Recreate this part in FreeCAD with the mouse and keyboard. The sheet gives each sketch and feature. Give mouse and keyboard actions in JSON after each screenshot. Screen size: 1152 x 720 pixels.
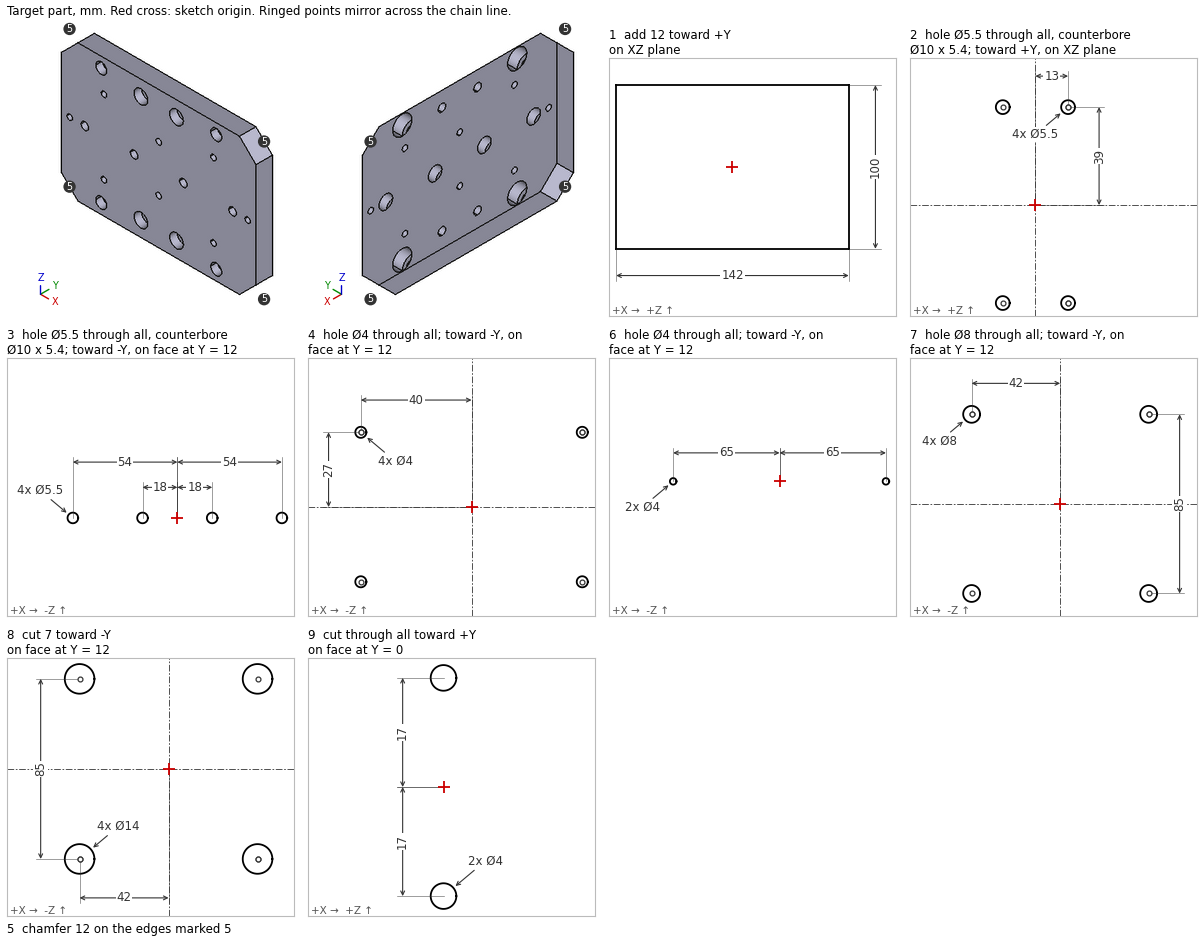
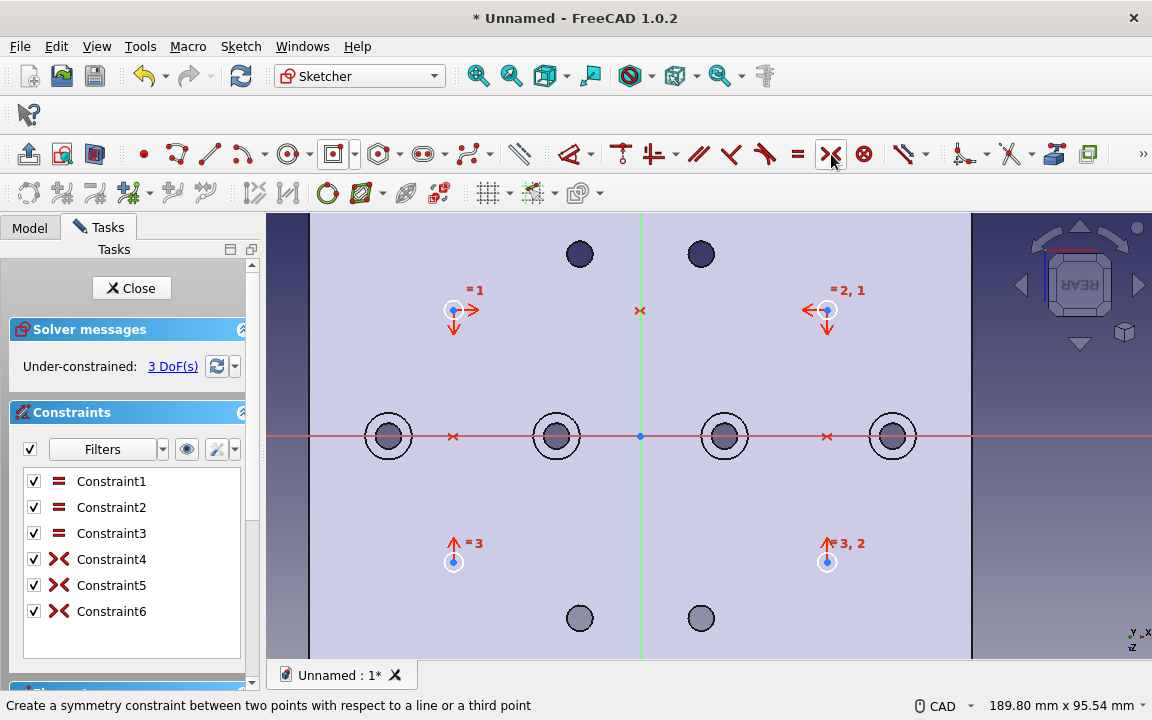
{"action": "left_click", "coordinate": [568, 154]}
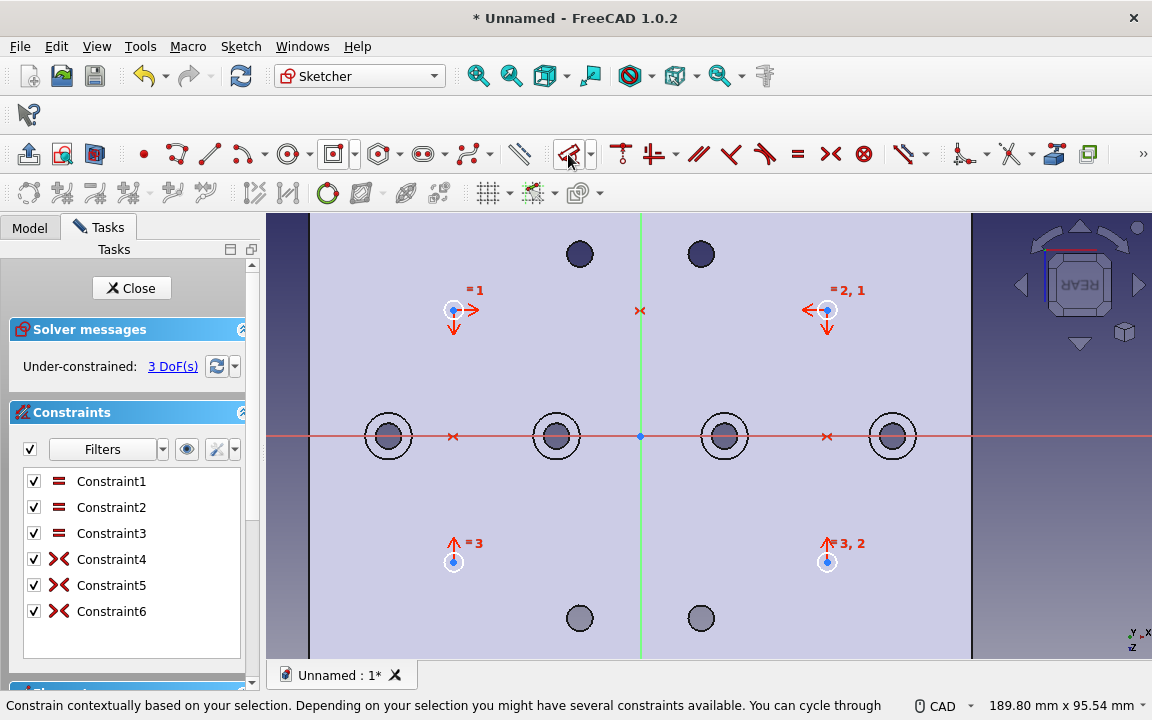
{"action": "scroll", "coordinate": [460, 303], "scroll_direction": "up", "scroll_amount": 4}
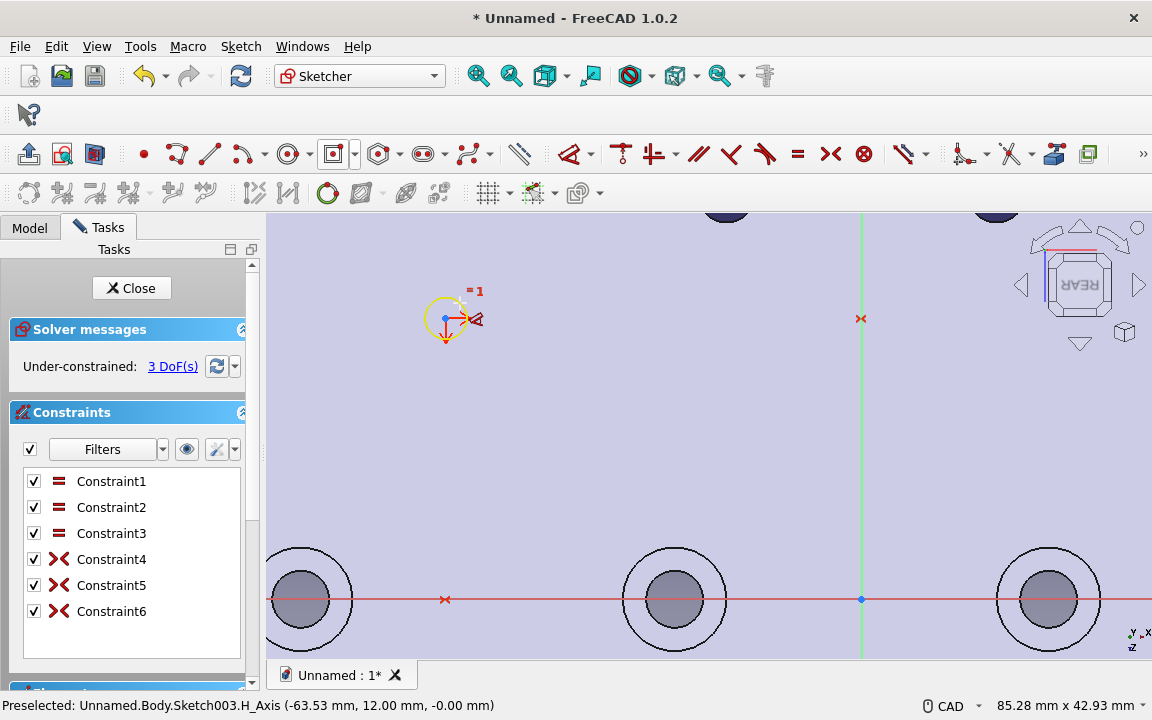
{"action": "left_click", "coordinate": [461, 304]}
{"action": "left_click", "coordinate": [484, 282]}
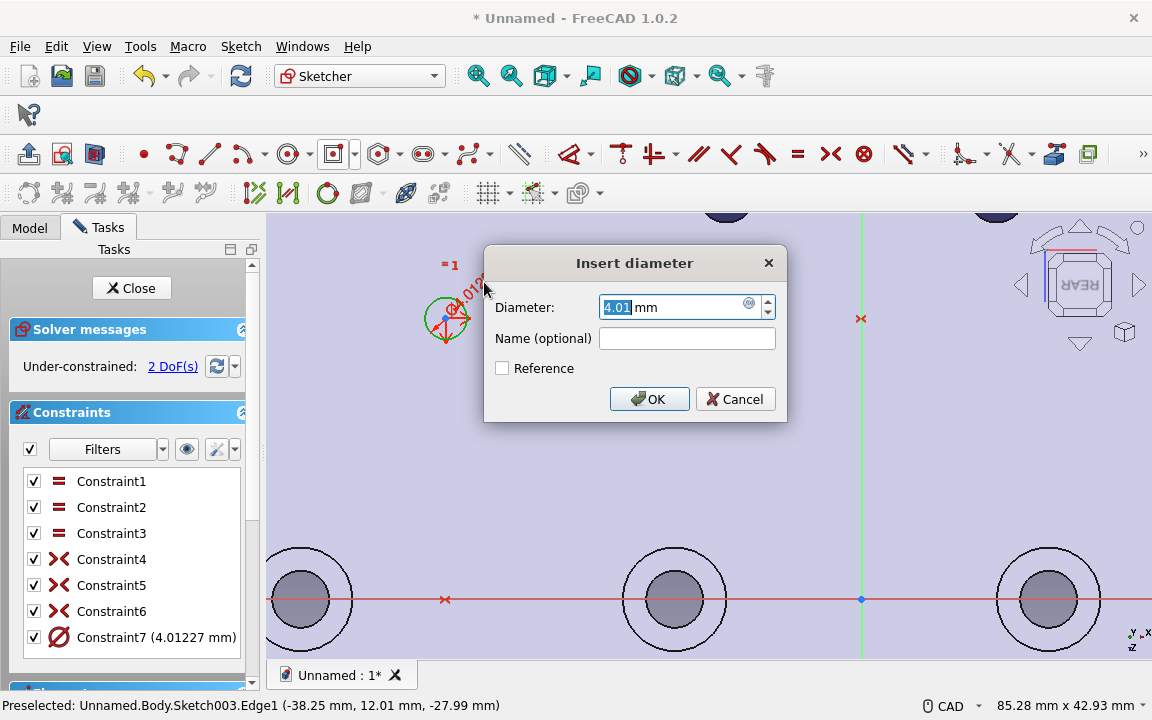
{"action": "type", "text": "4"}
{"action": "key", "text": "Return"}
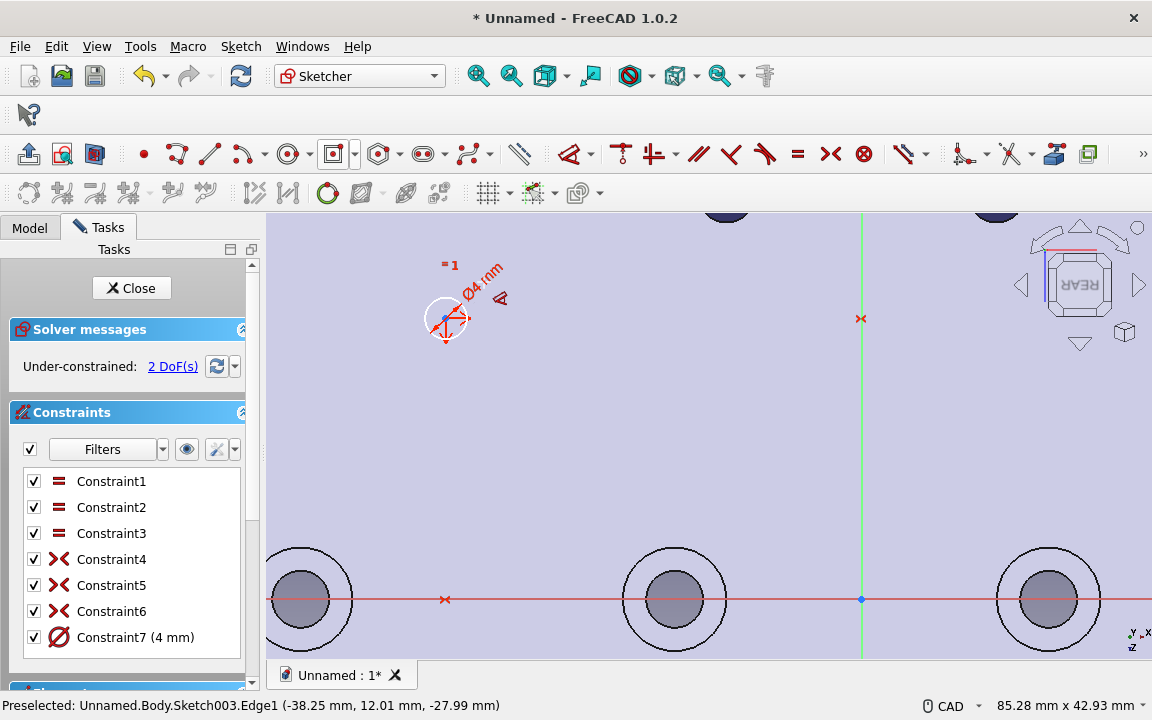
{"action": "left_click", "coordinate": [446, 318]}
{"action": "left_click", "coordinate": [654, 284]}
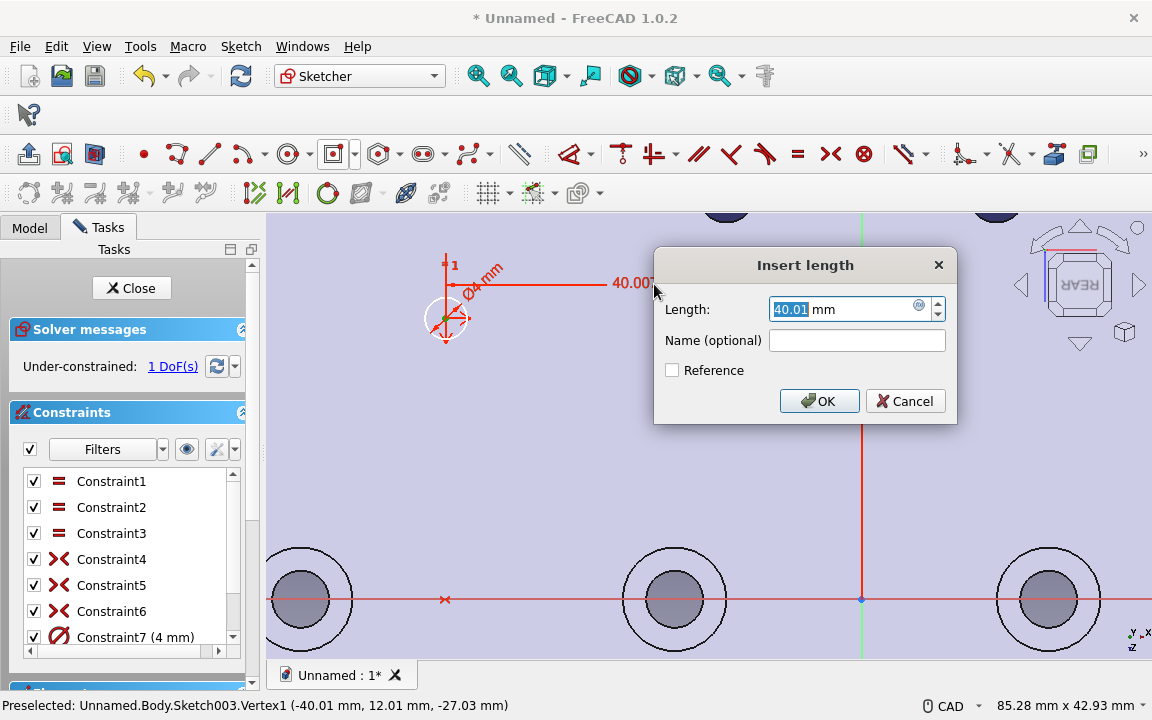
{"action": "type", "text": "40"}
{"action": "key", "text": "Return"}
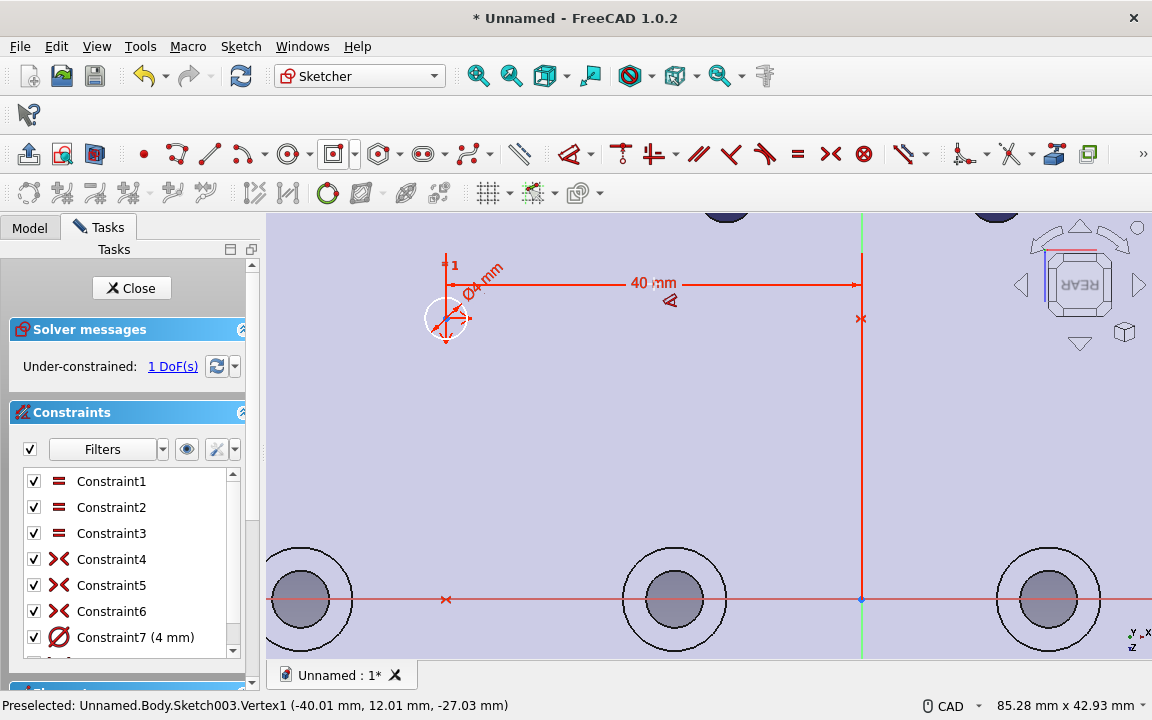
{"action": "left_click", "coordinate": [446, 318]}
{"action": "left_click", "coordinate": [412, 459]}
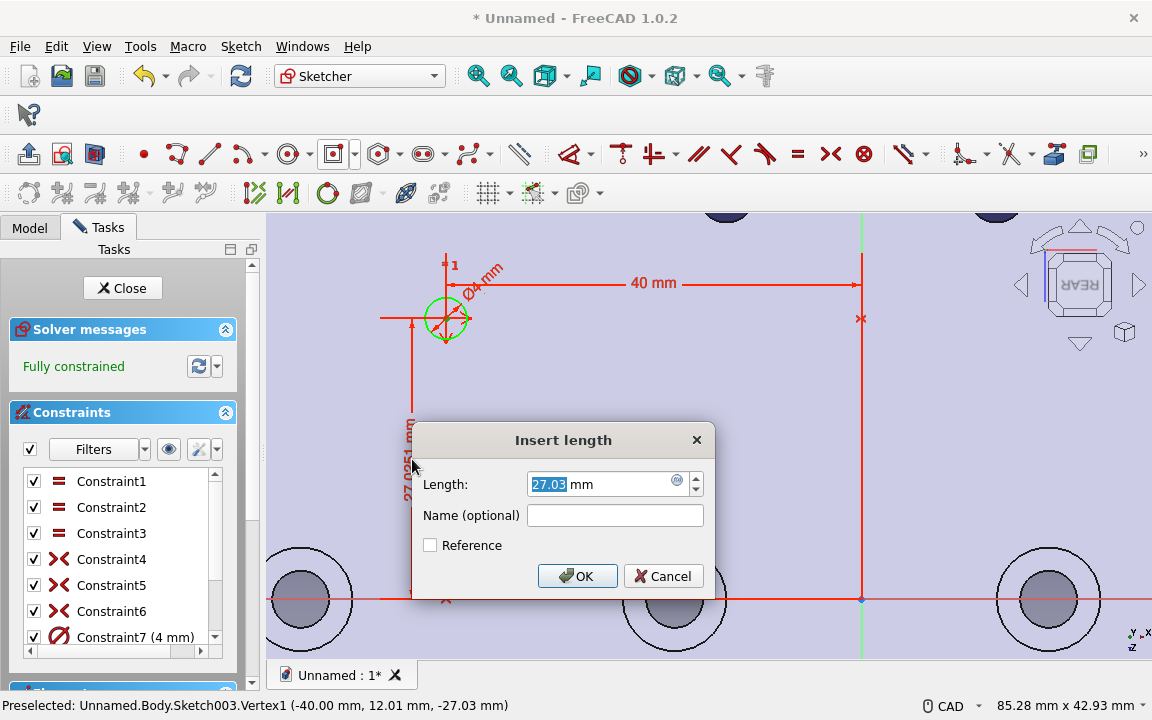
{"action": "type", "text": "27"}
{"action": "key", "text": "Return"}
{"action": "key", "text": "Escape"}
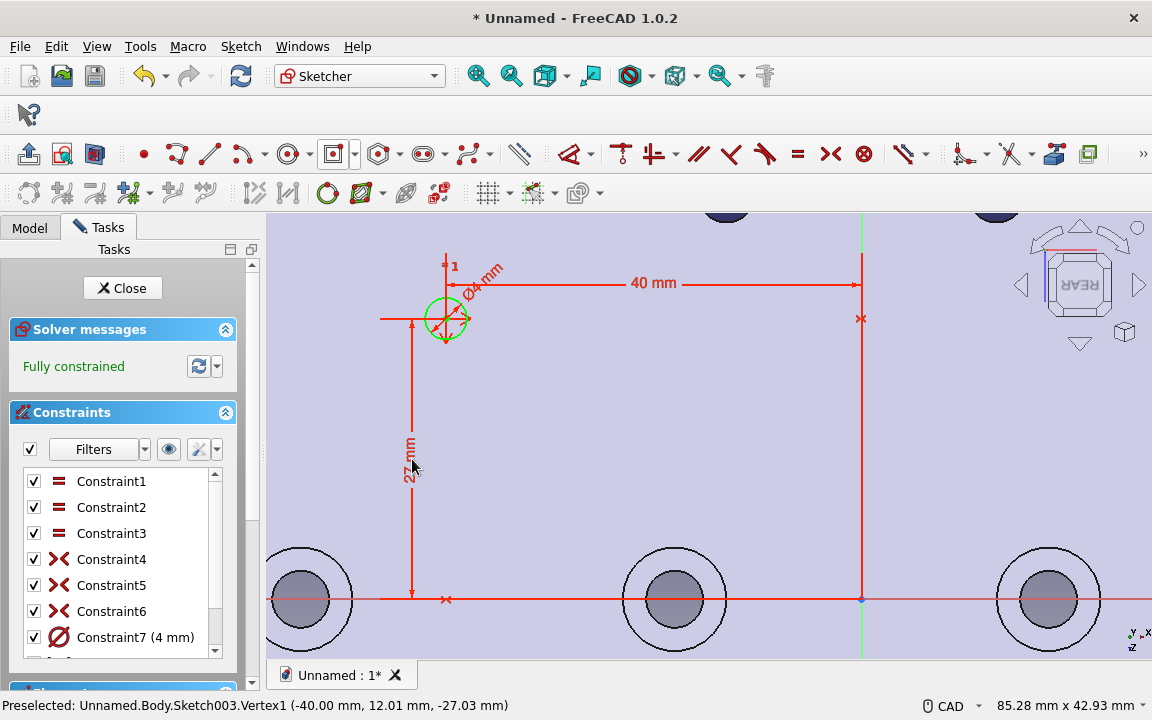
{"action": "left_click", "coordinate": [123, 288]}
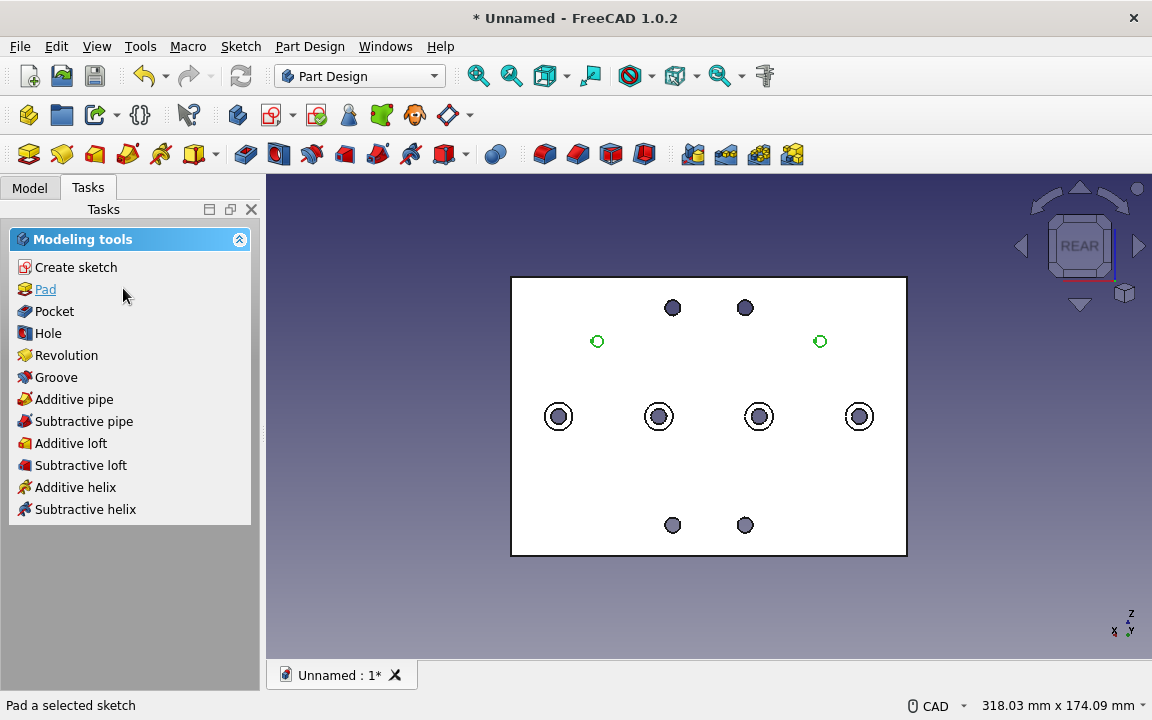
{"action": "left_click", "coordinate": [279, 154]}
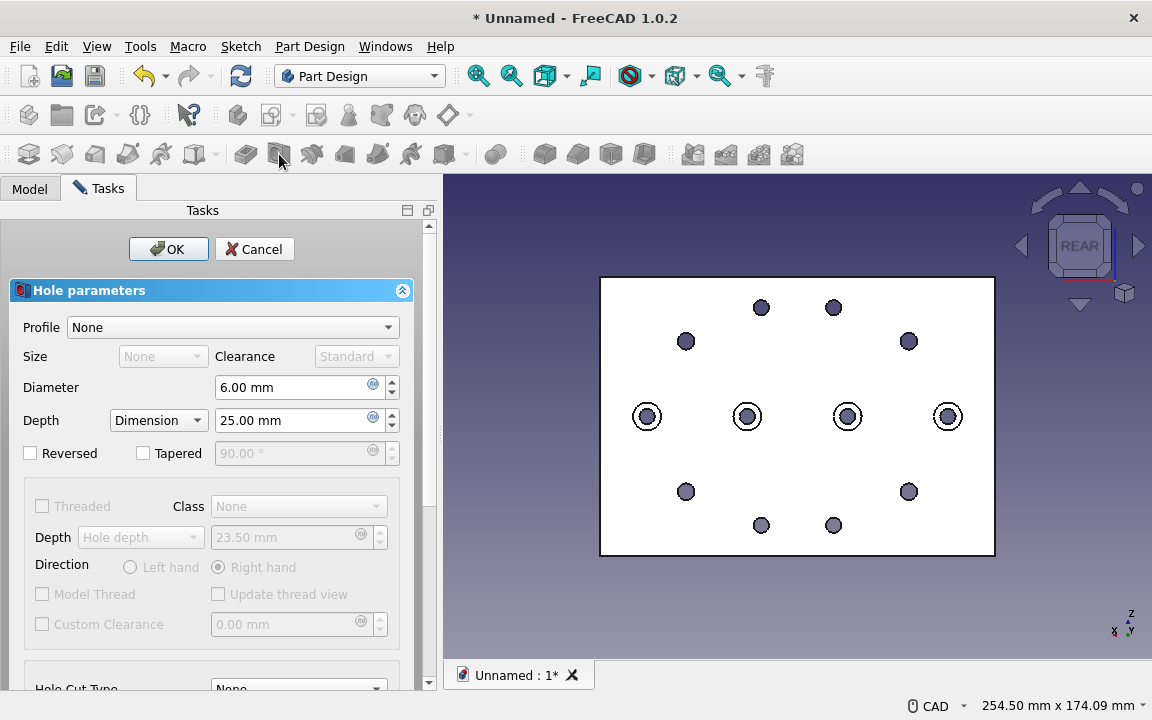
{"action": "triple_click", "coordinate": [300, 388]}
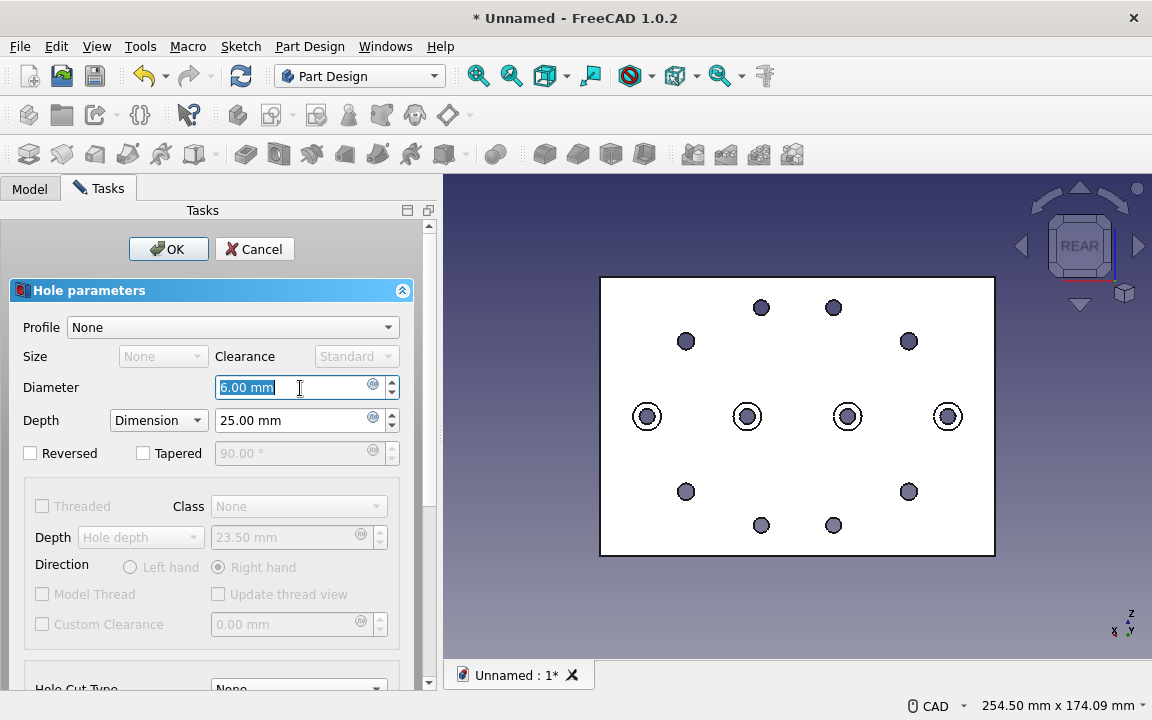
{"action": "type", "text": "4"}
{"action": "key", "text": "Tab"}